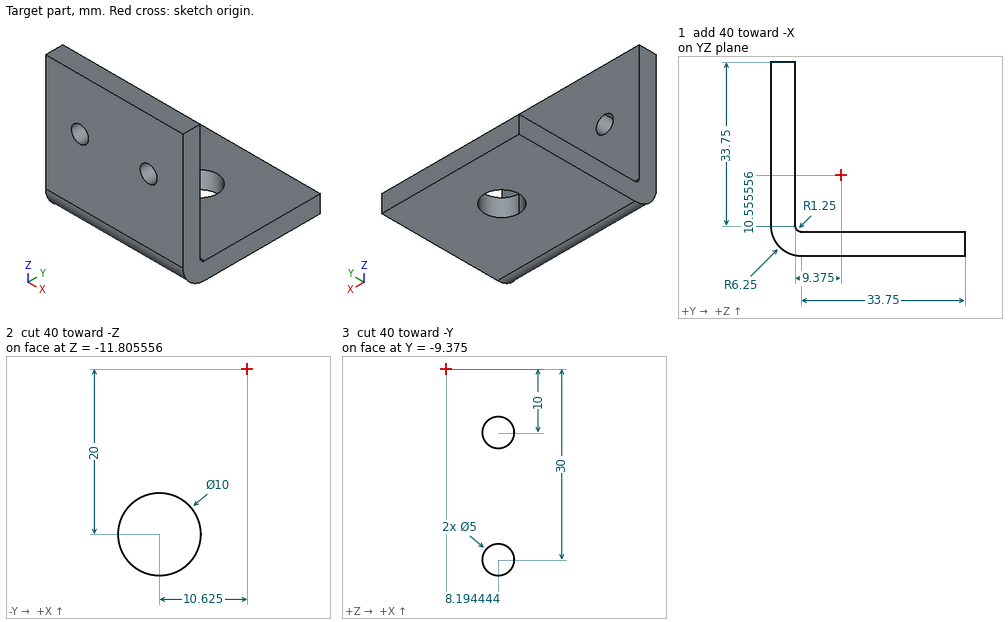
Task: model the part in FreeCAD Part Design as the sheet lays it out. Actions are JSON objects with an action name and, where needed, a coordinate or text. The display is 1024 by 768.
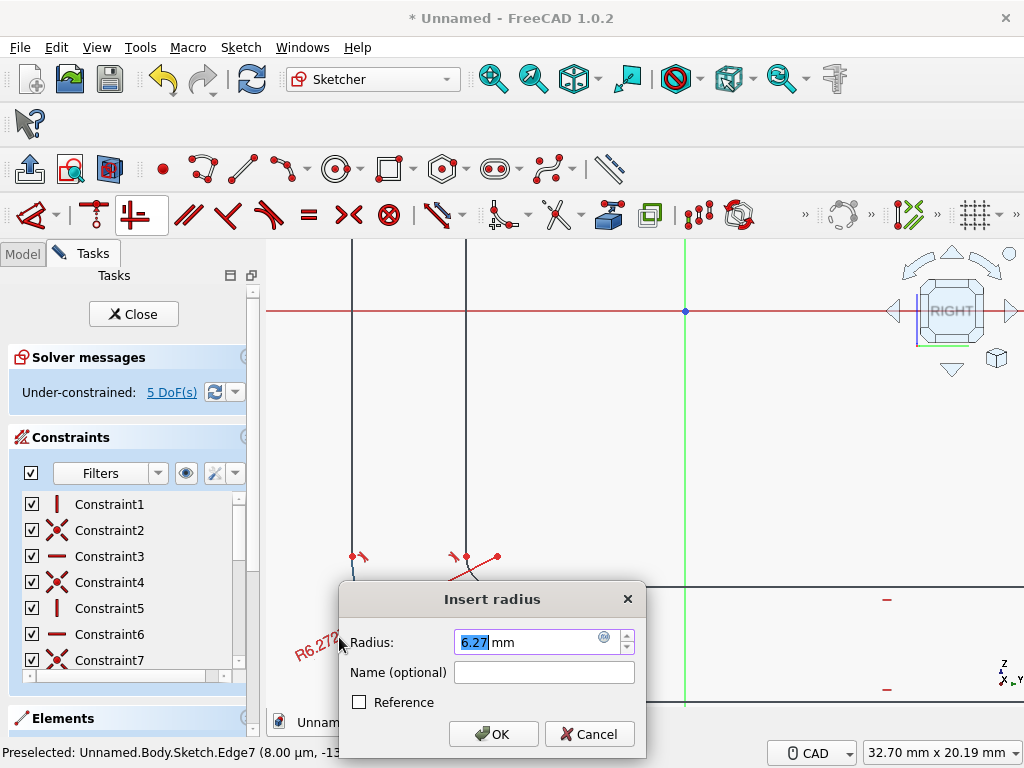
{"action": "type", "text": "6.25"}
{"action": "key", "text": "Return"}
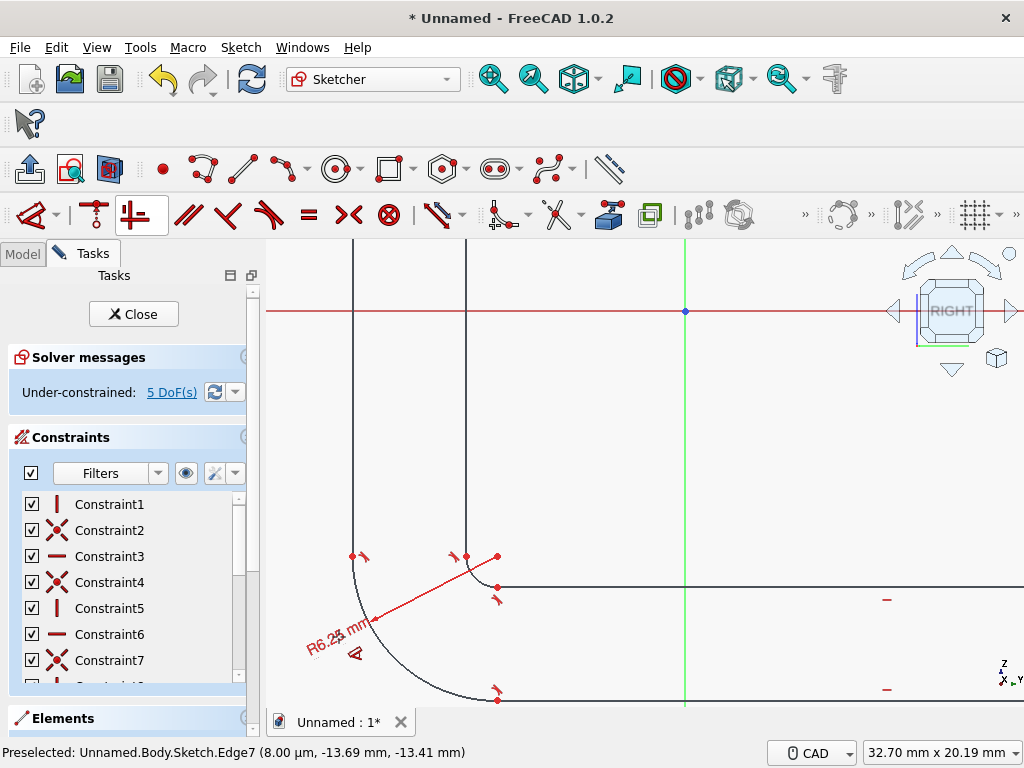
{"action": "scroll", "coordinate": [470, 570], "scroll_direction": "up", "scroll_amount": 2}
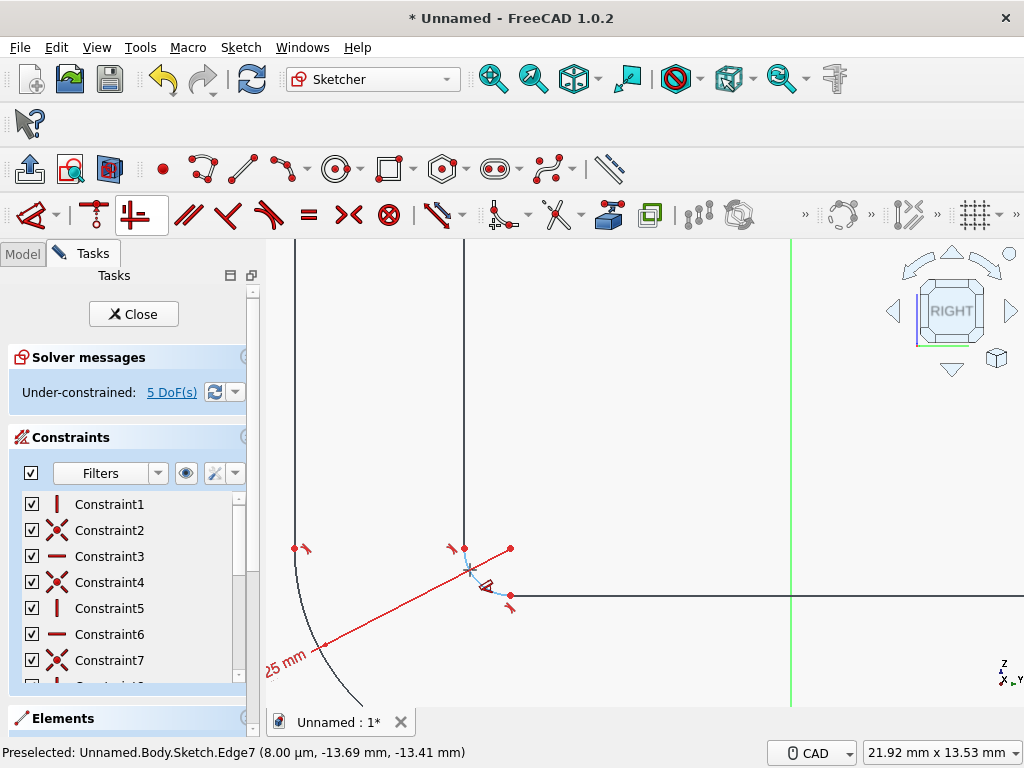
{"action": "left_click", "coordinate": [469, 570]}
{"action": "left_click", "coordinate": [440, 584]}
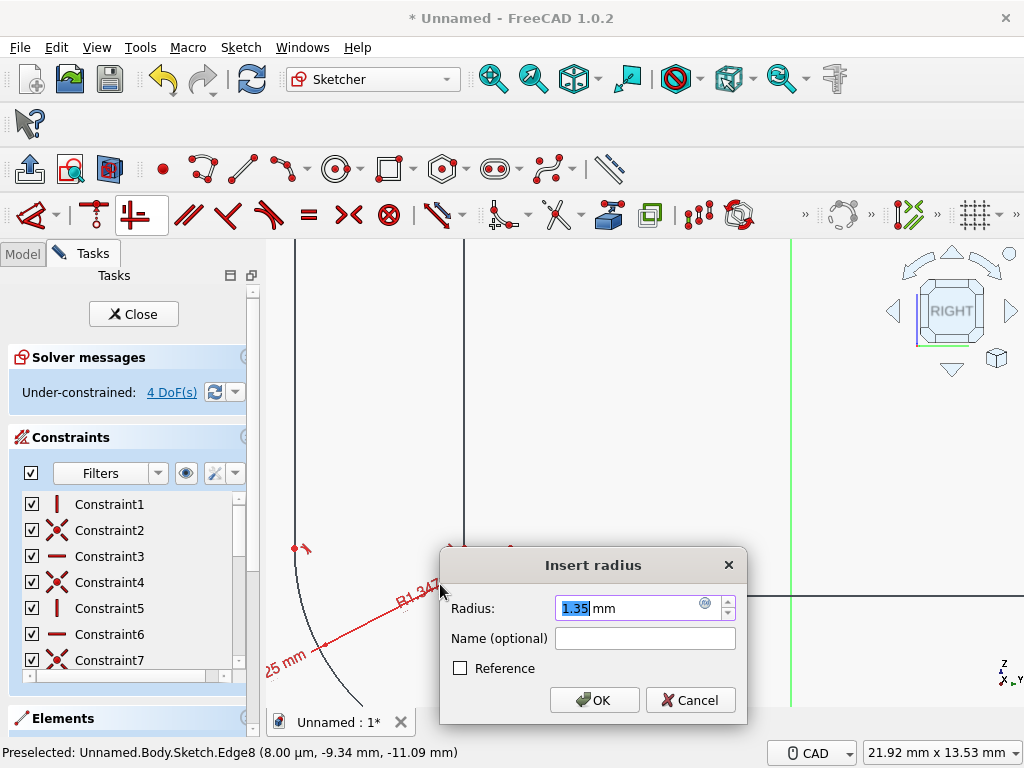
{"action": "type", "text": "1.25"}
{"action": "key", "text": "Return"}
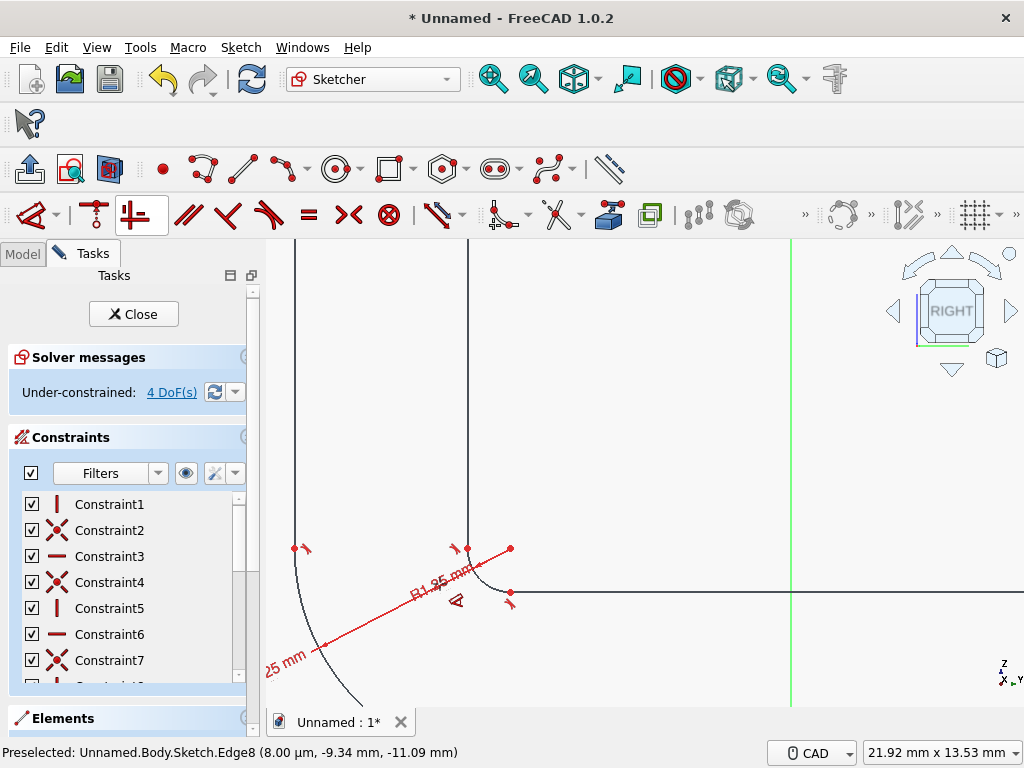
{"action": "scroll", "coordinate": [473, 574], "scroll_direction": "down", "scroll_amount": 8}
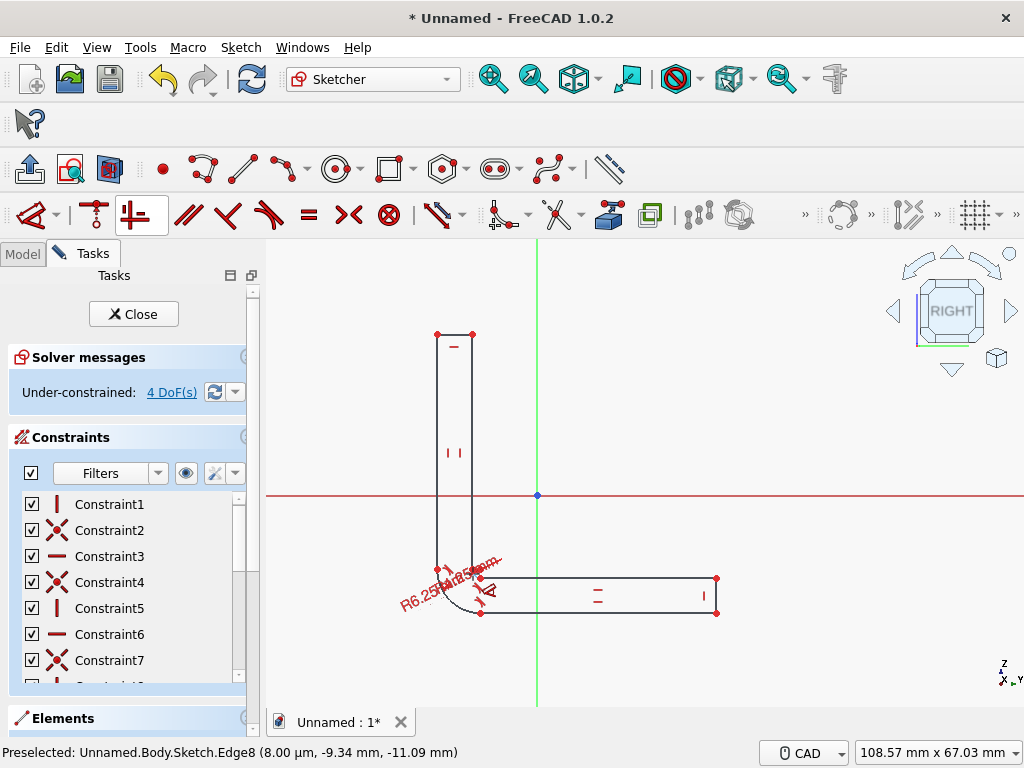
{"action": "left_click", "coordinate": [472, 523]}
{"action": "left_click", "coordinate": [506, 452]}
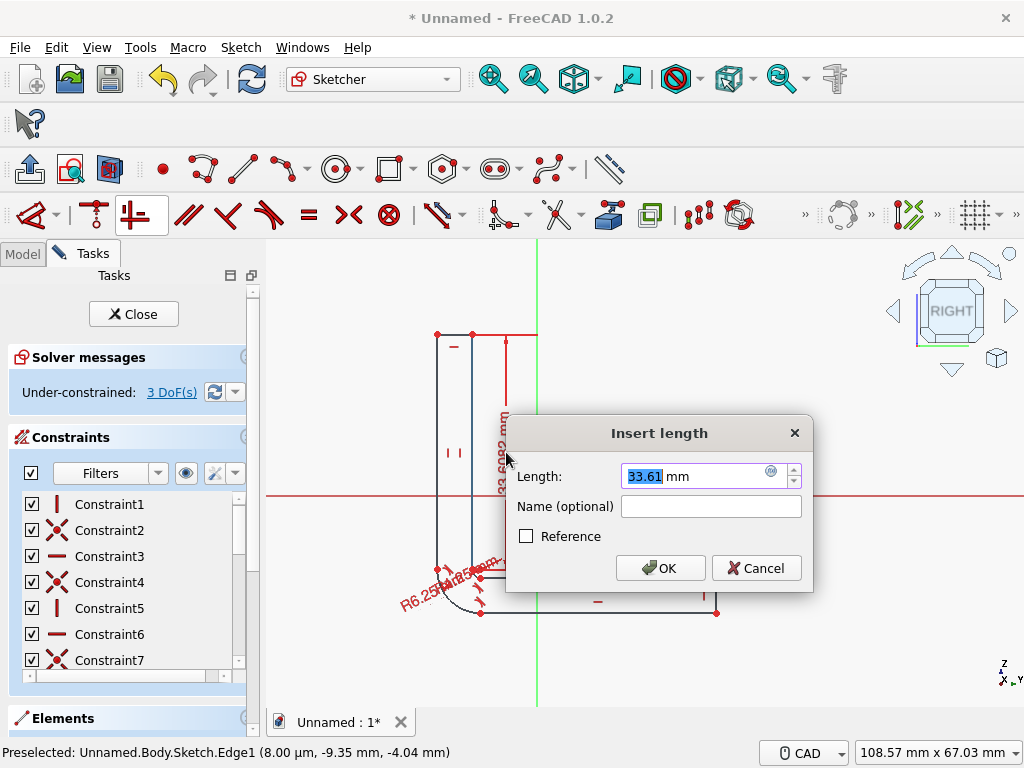
{"action": "type", "text": "33.75"}
{"action": "key", "text": "Return"}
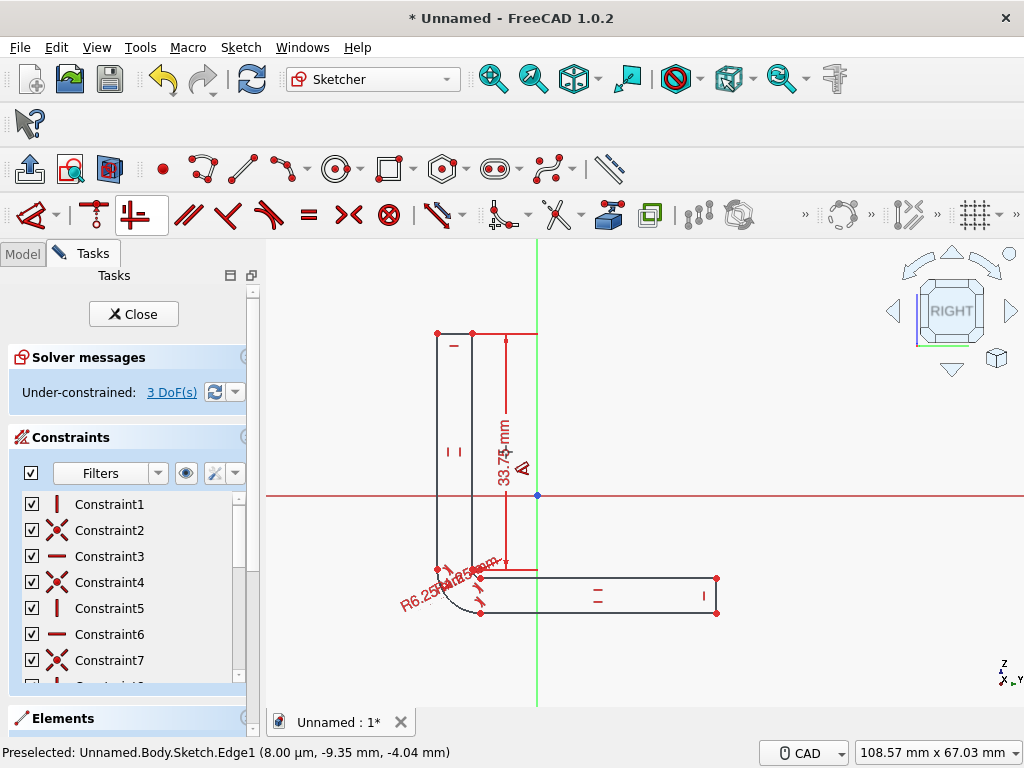
{"action": "left_click", "coordinate": [551, 613]}
{"action": "left_click", "coordinate": [598, 647]}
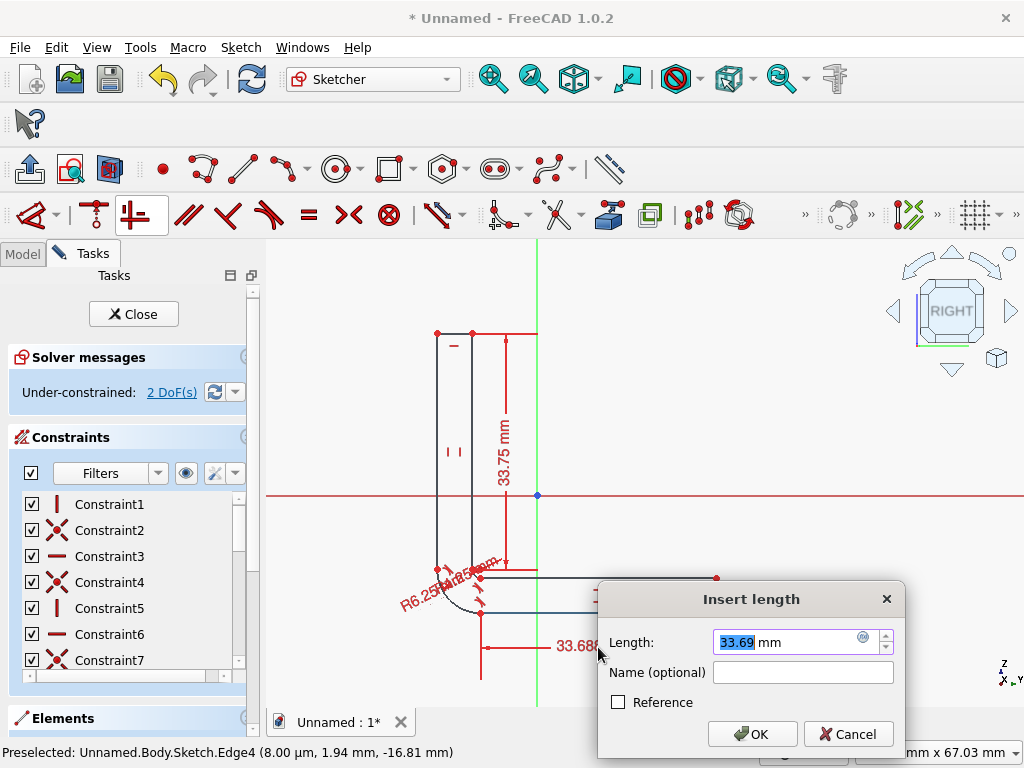
{"action": "type", "text": "33.75"}
{"action": "key", "text": "Return"}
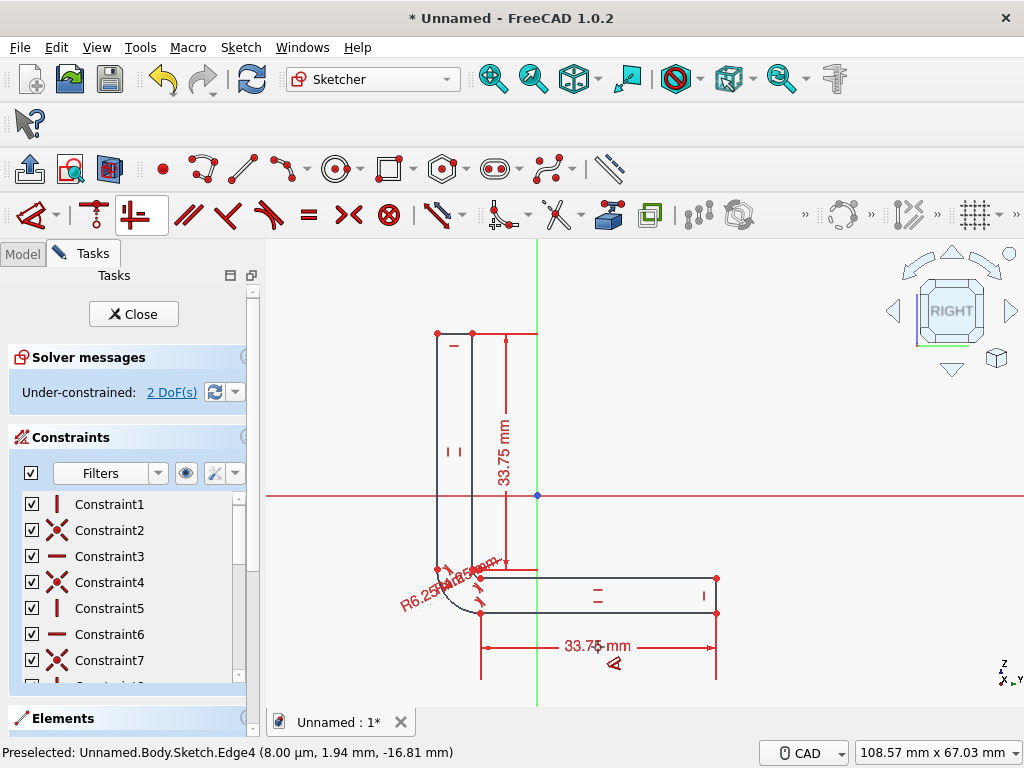
{"action": "scroll", "coordinate": [472, 570], "scroll_direction": "up", "scroll_amount": 2}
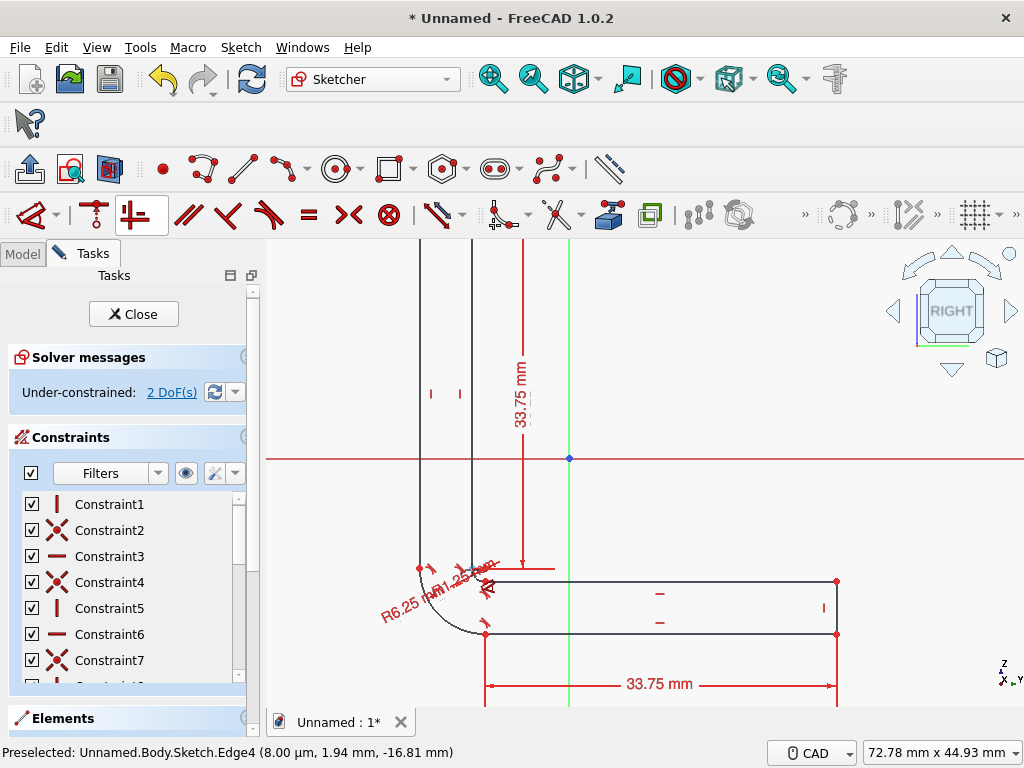
{"action": "left_click", "coordinate": [472, 569]}
{"action": "left_click", "coordinate": [521, 603]}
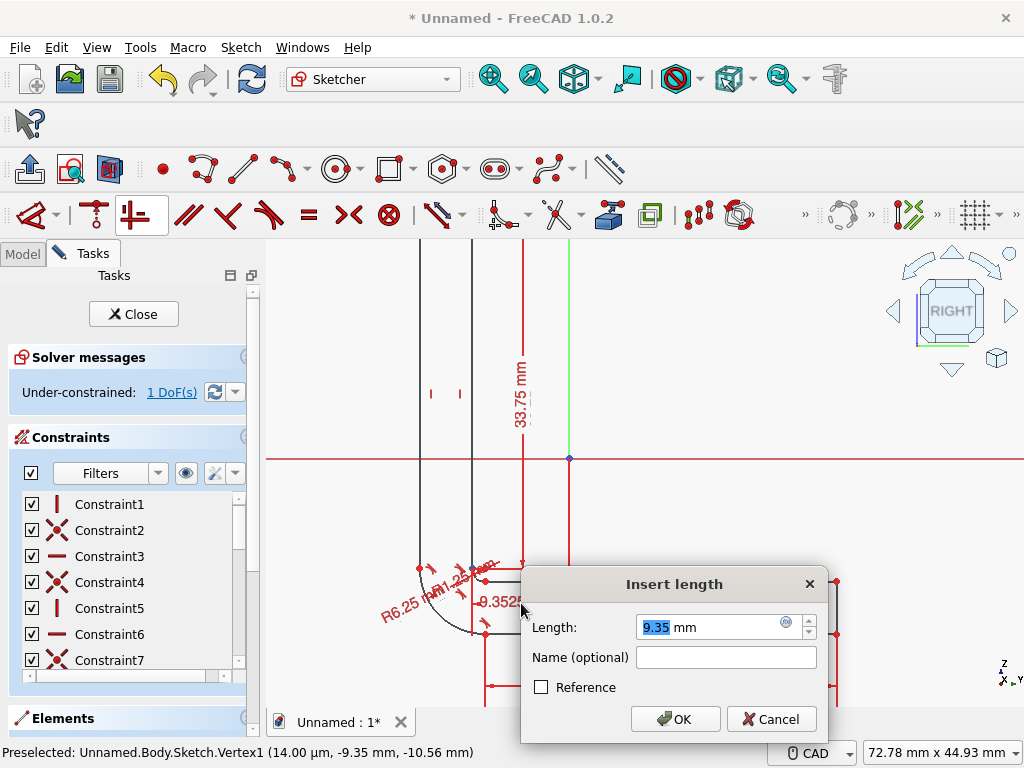
{"action": "type", "text": "9.375"}
{"action": "key", "text": "Return"}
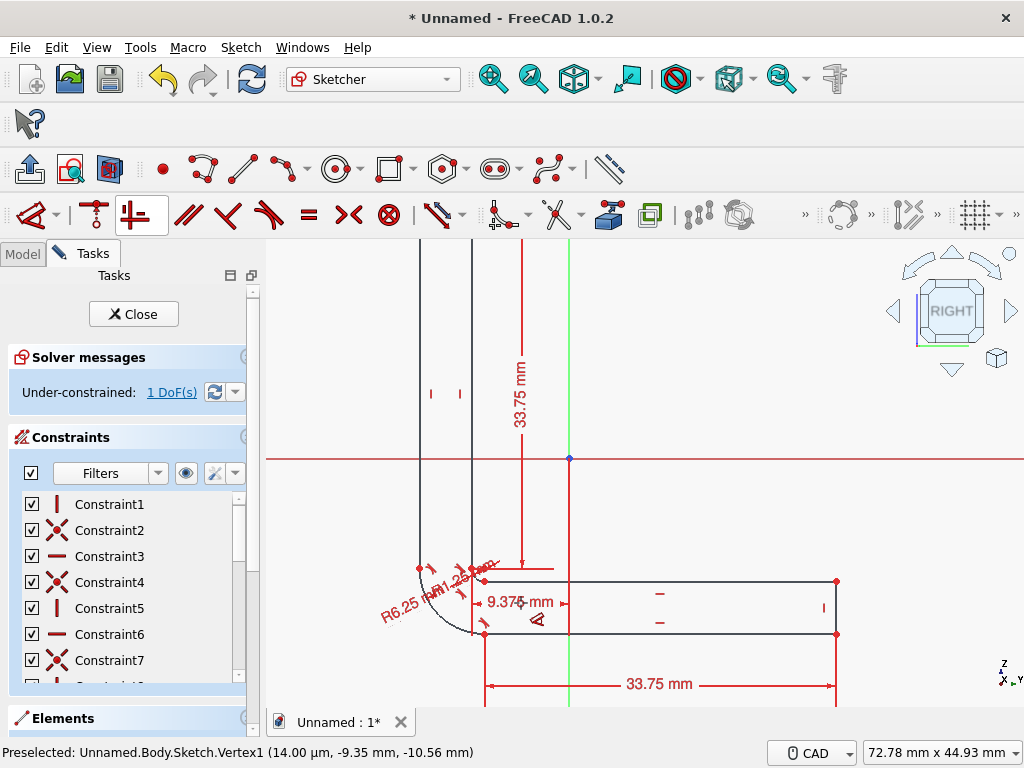
{"action": "left_click", "coordinate": [472, 569]}
{"action": "left_click", "coordinate": [438, 514]}